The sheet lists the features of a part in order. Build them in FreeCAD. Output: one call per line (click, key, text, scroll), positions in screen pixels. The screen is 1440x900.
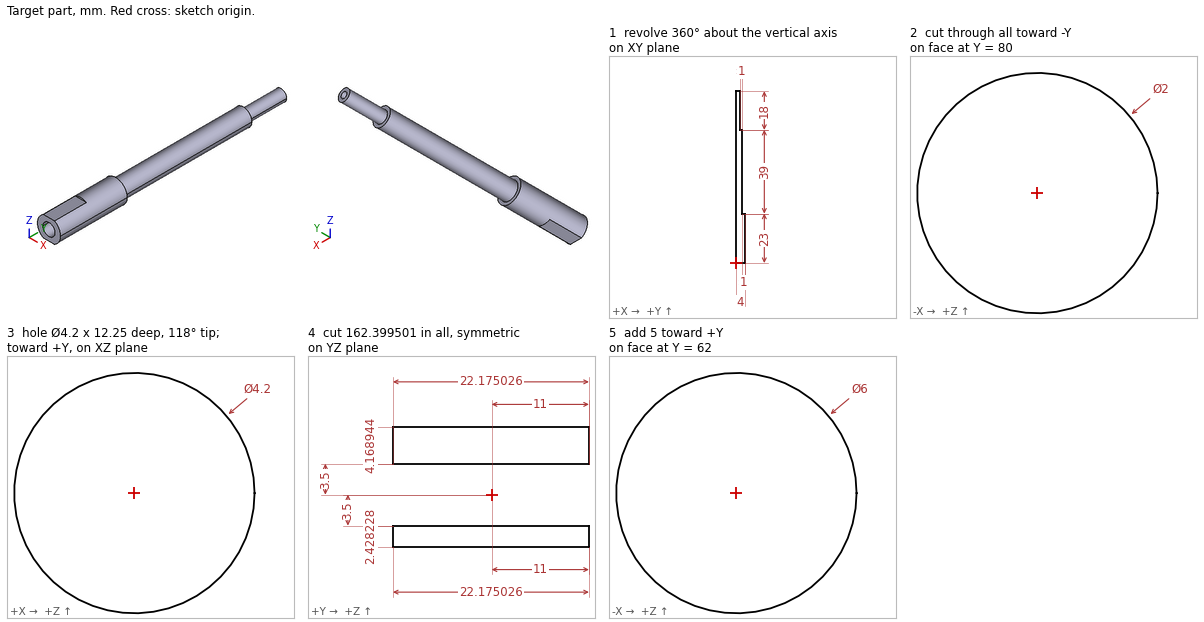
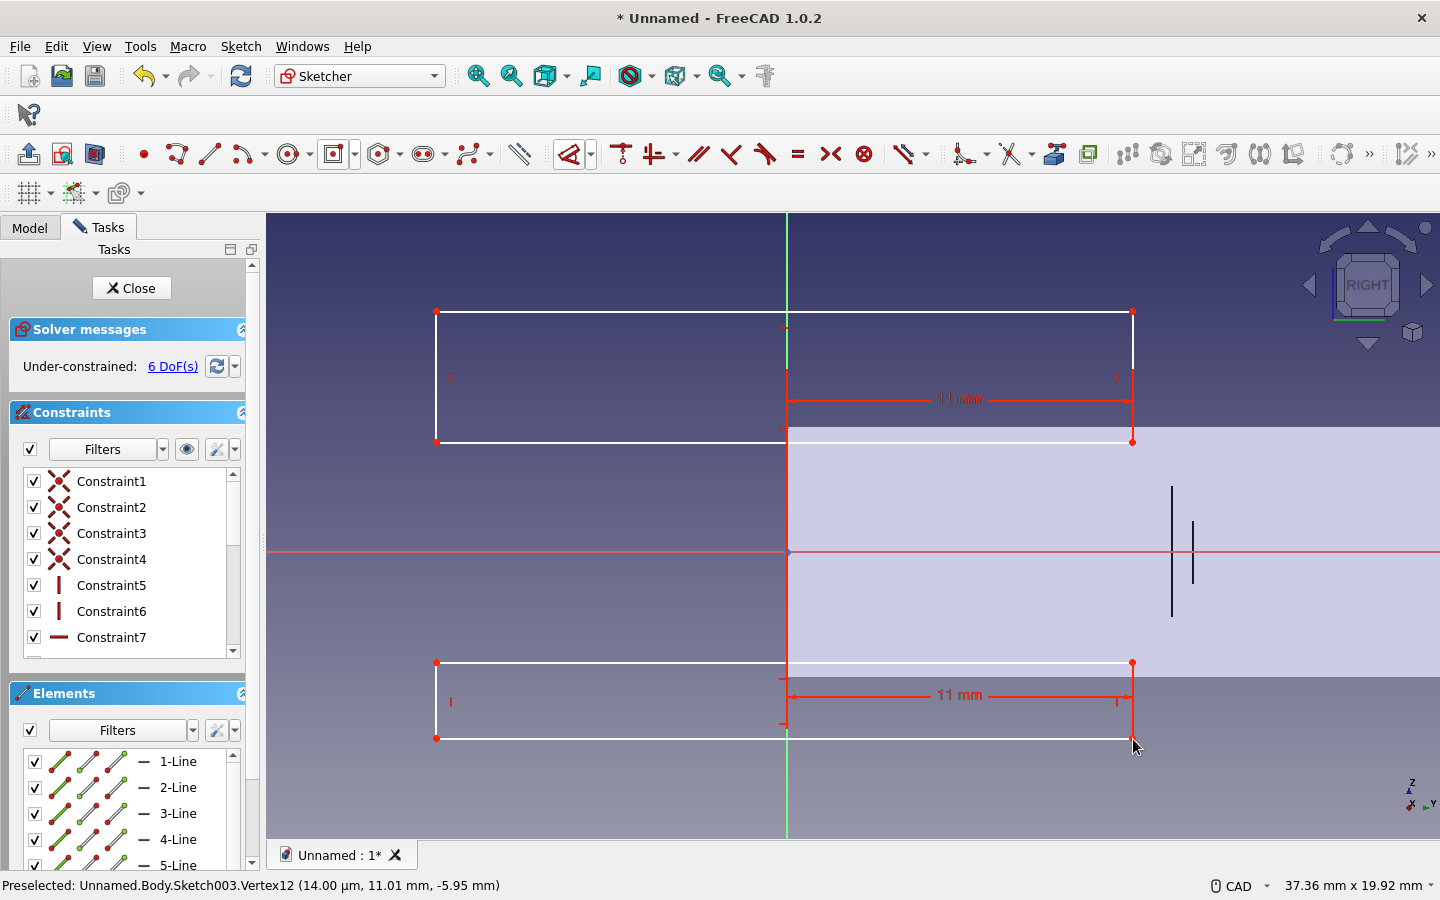
click(436, 443)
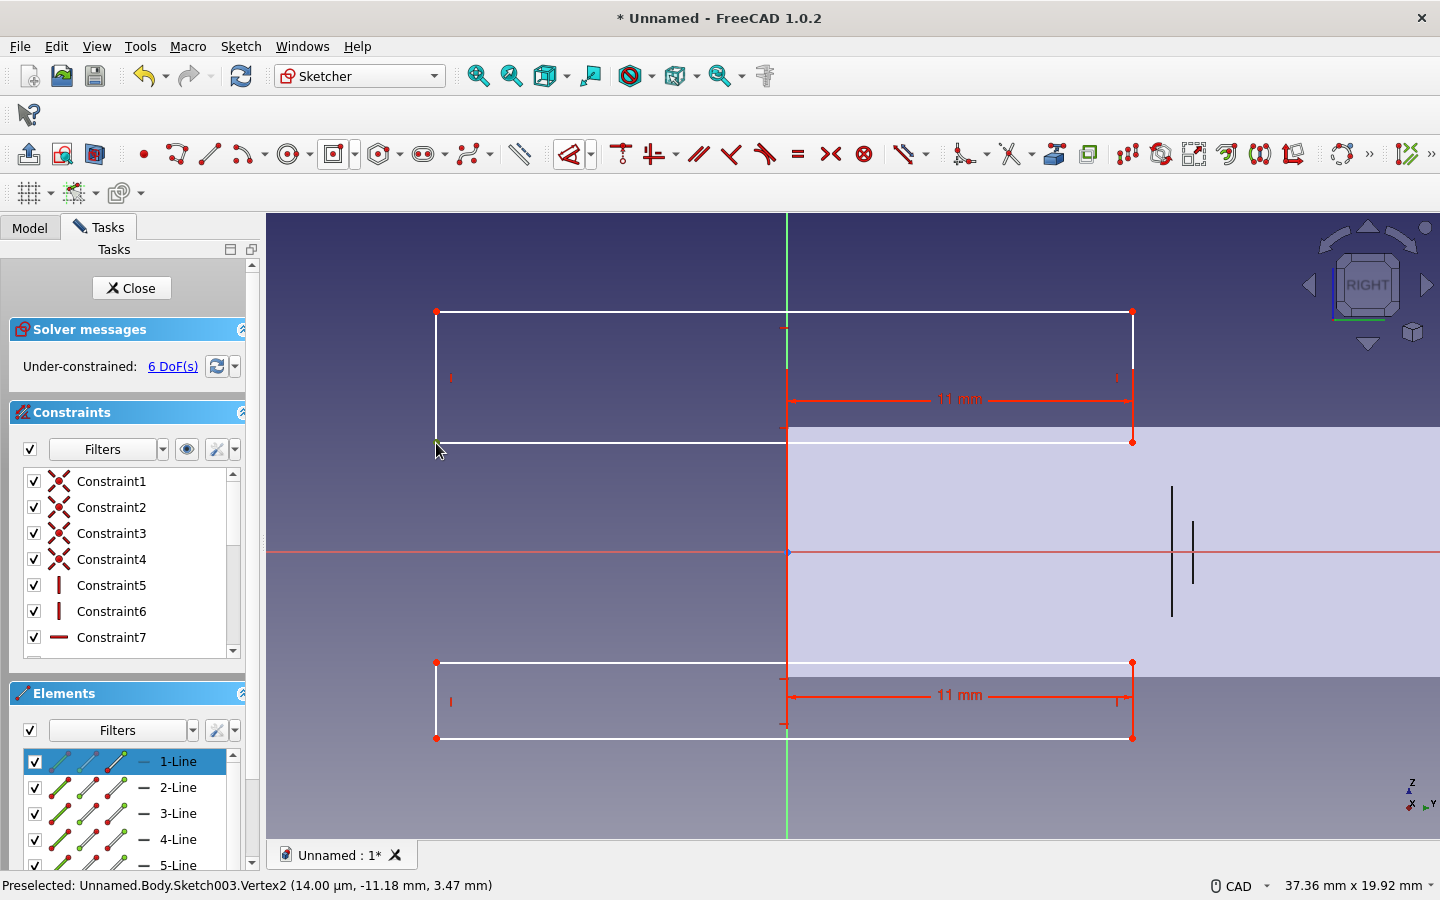
key(i)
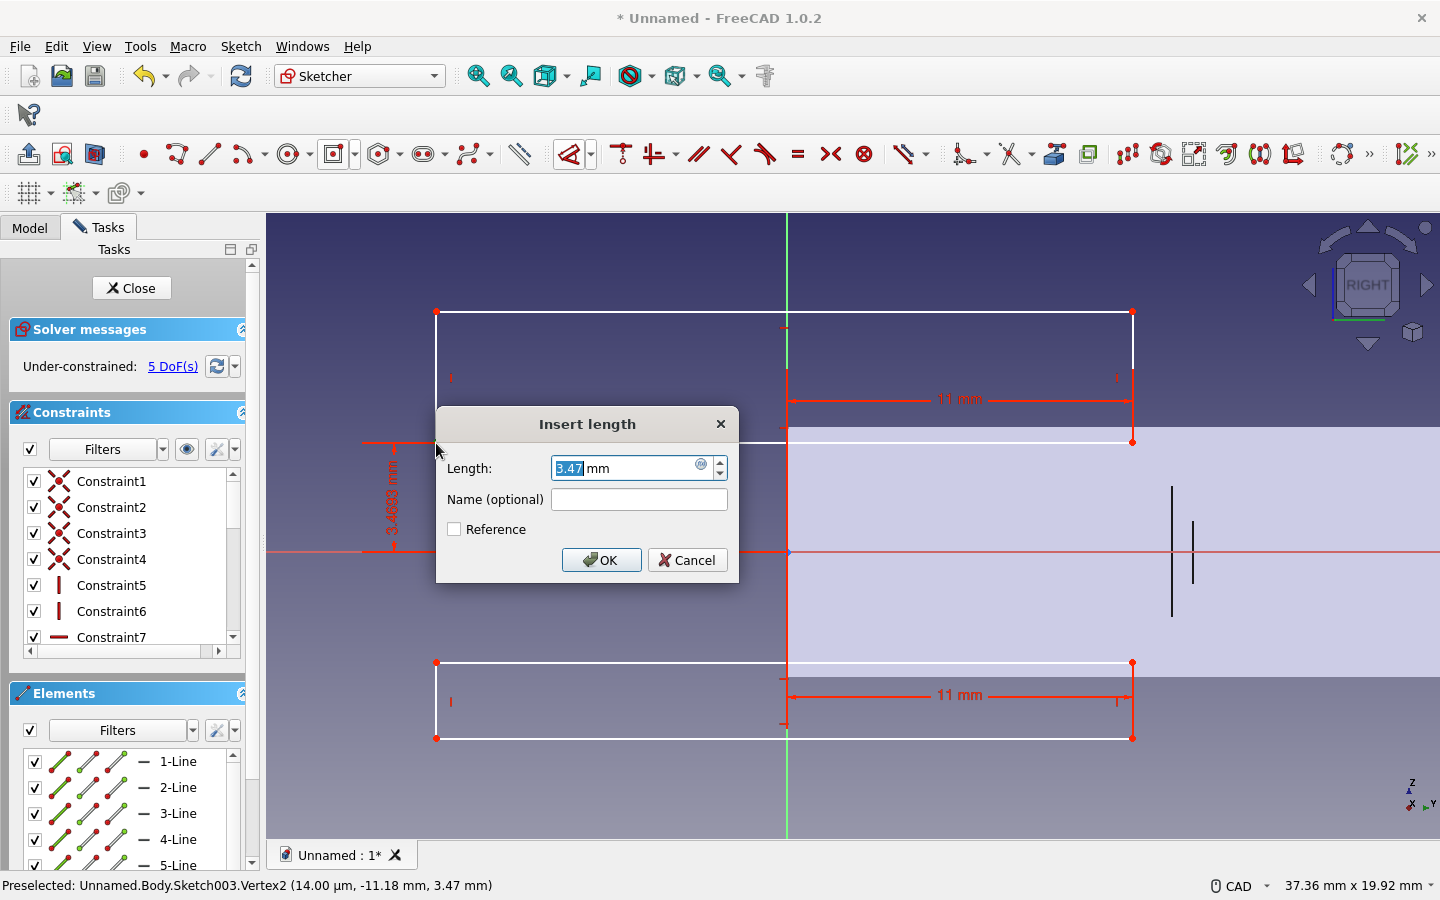
text(3.5)
key(Return)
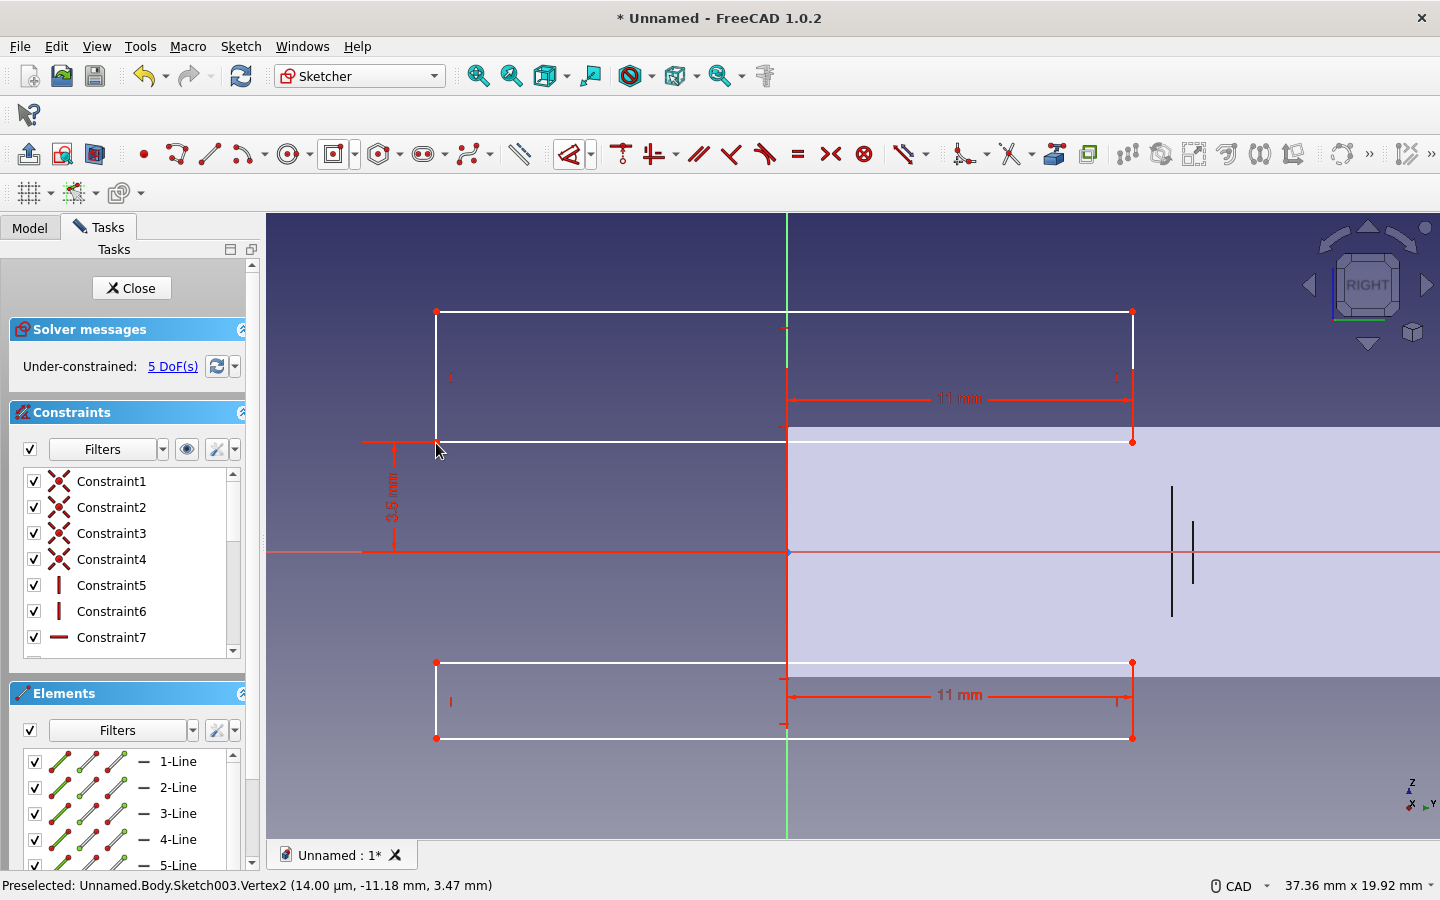
click(436, 663)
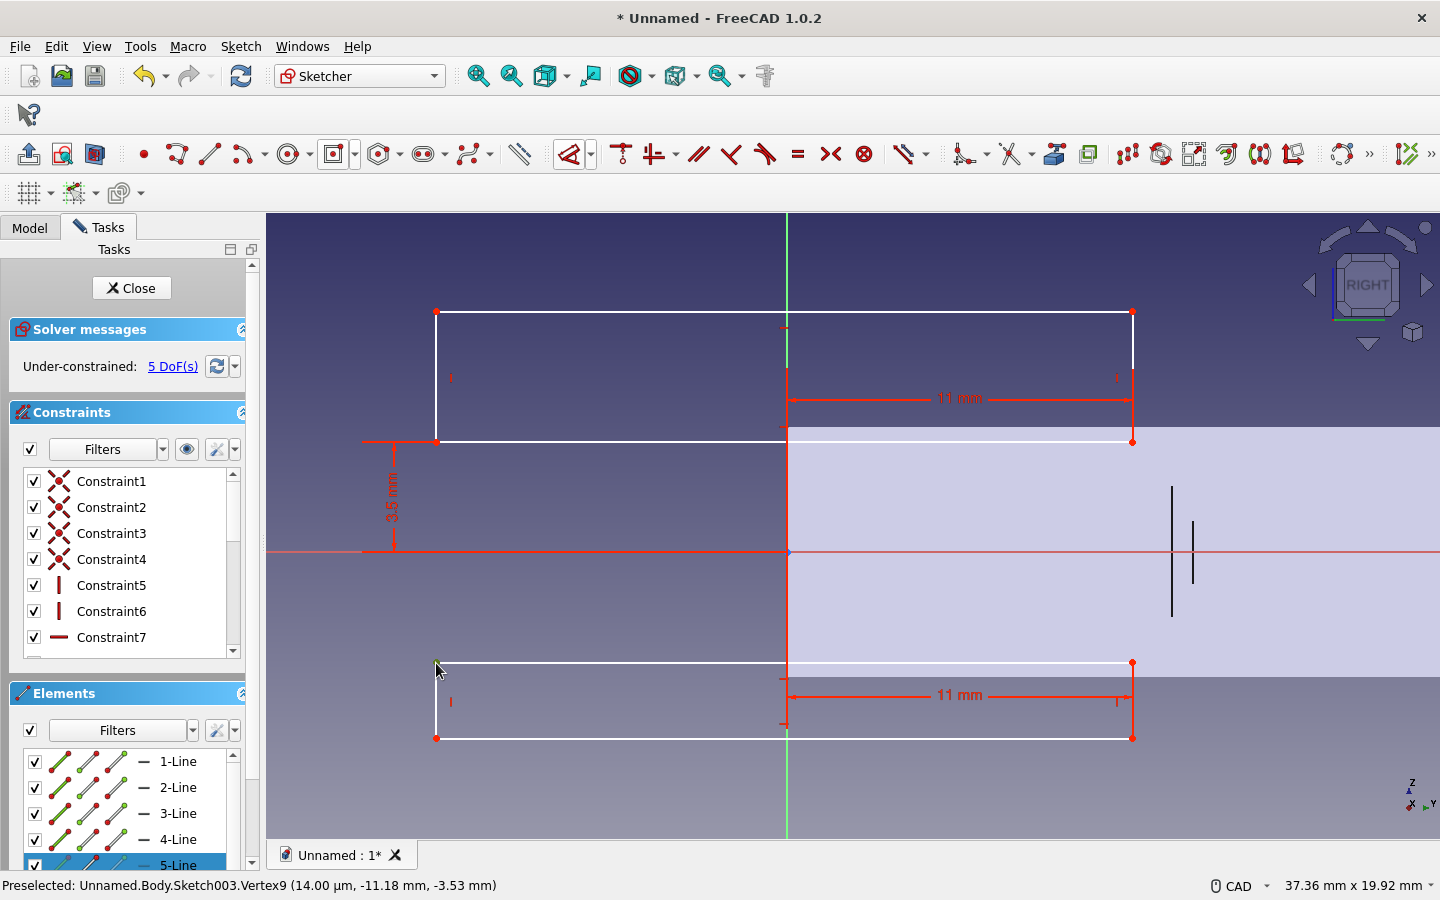
key(i)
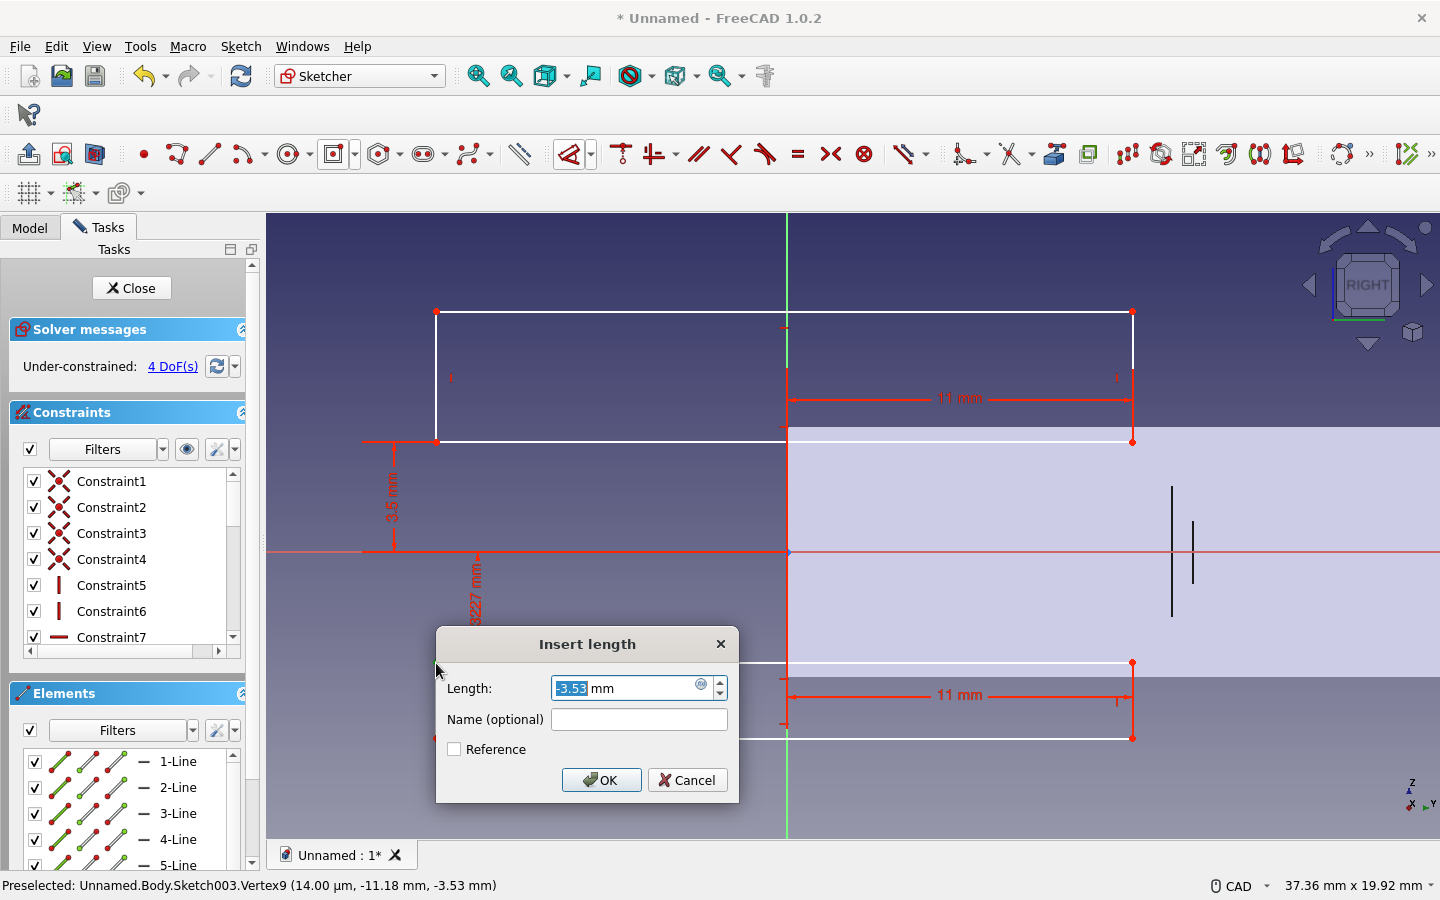
text(-3.5)
key(Return)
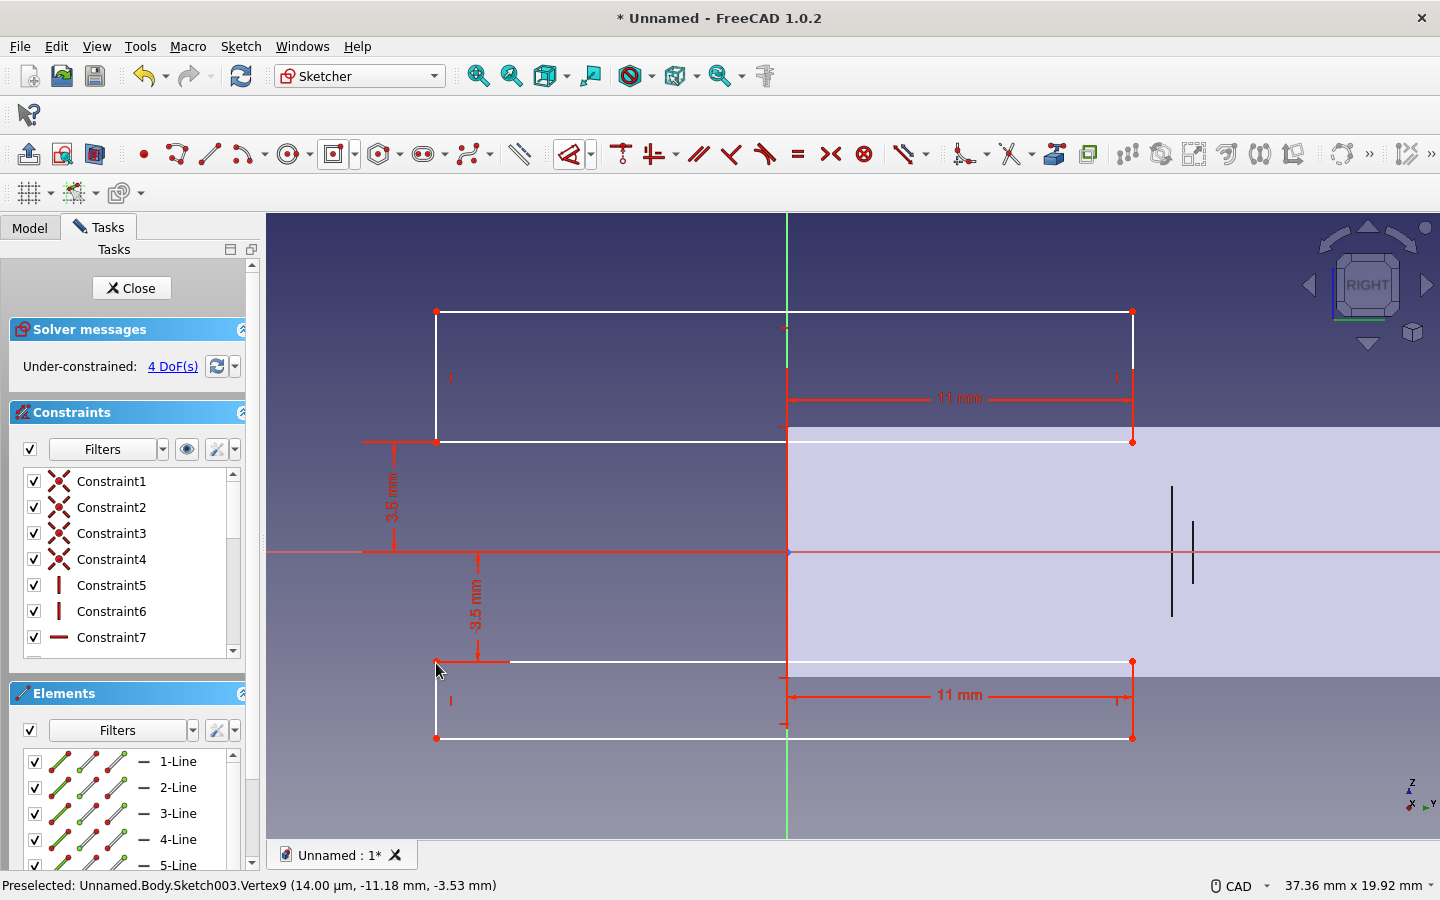
click(436, 351)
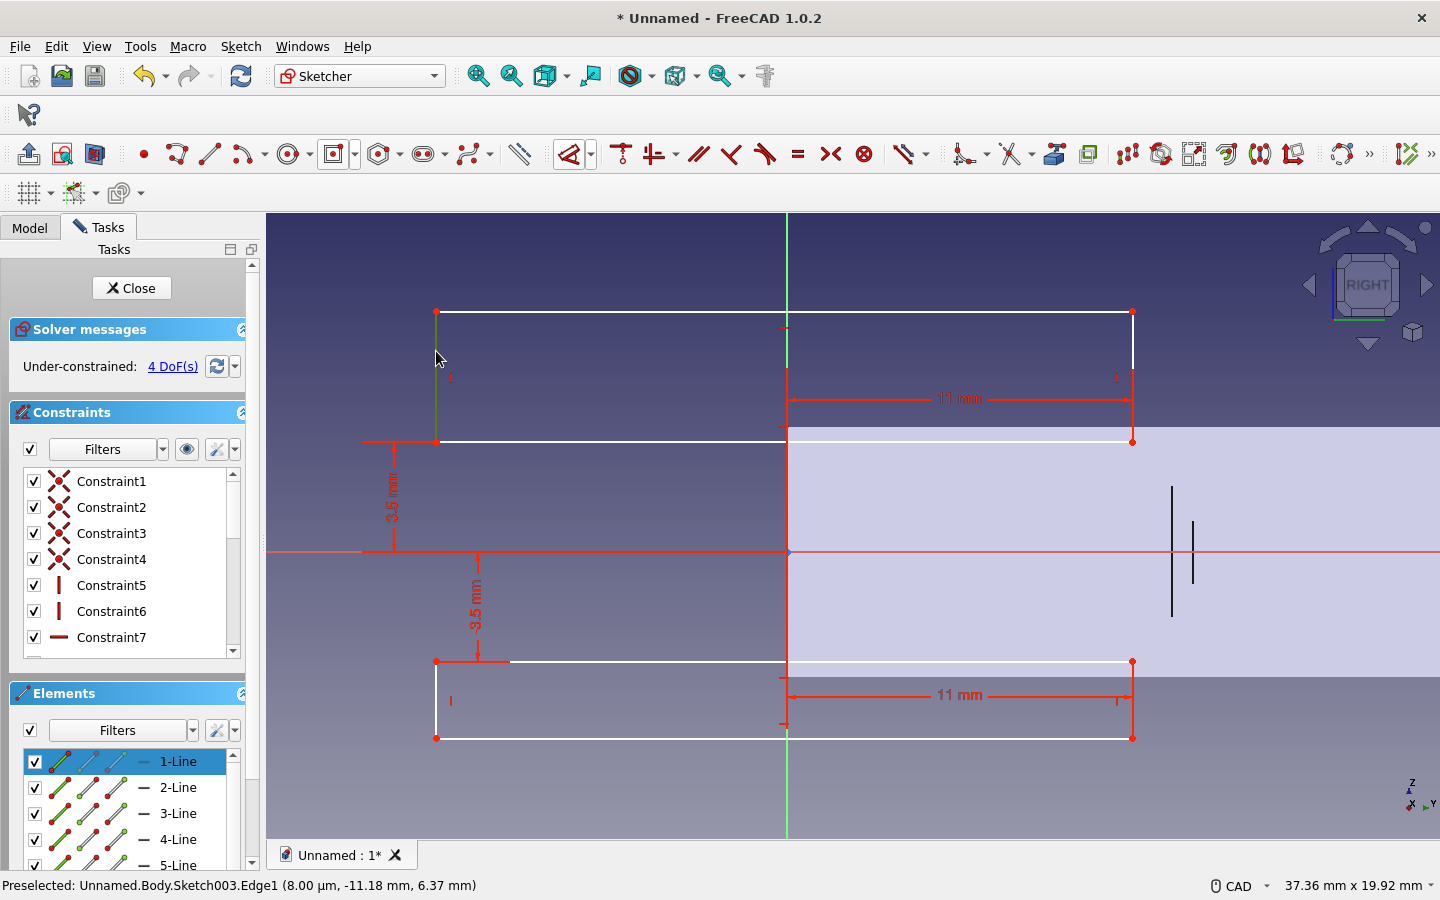
click(590, 154)